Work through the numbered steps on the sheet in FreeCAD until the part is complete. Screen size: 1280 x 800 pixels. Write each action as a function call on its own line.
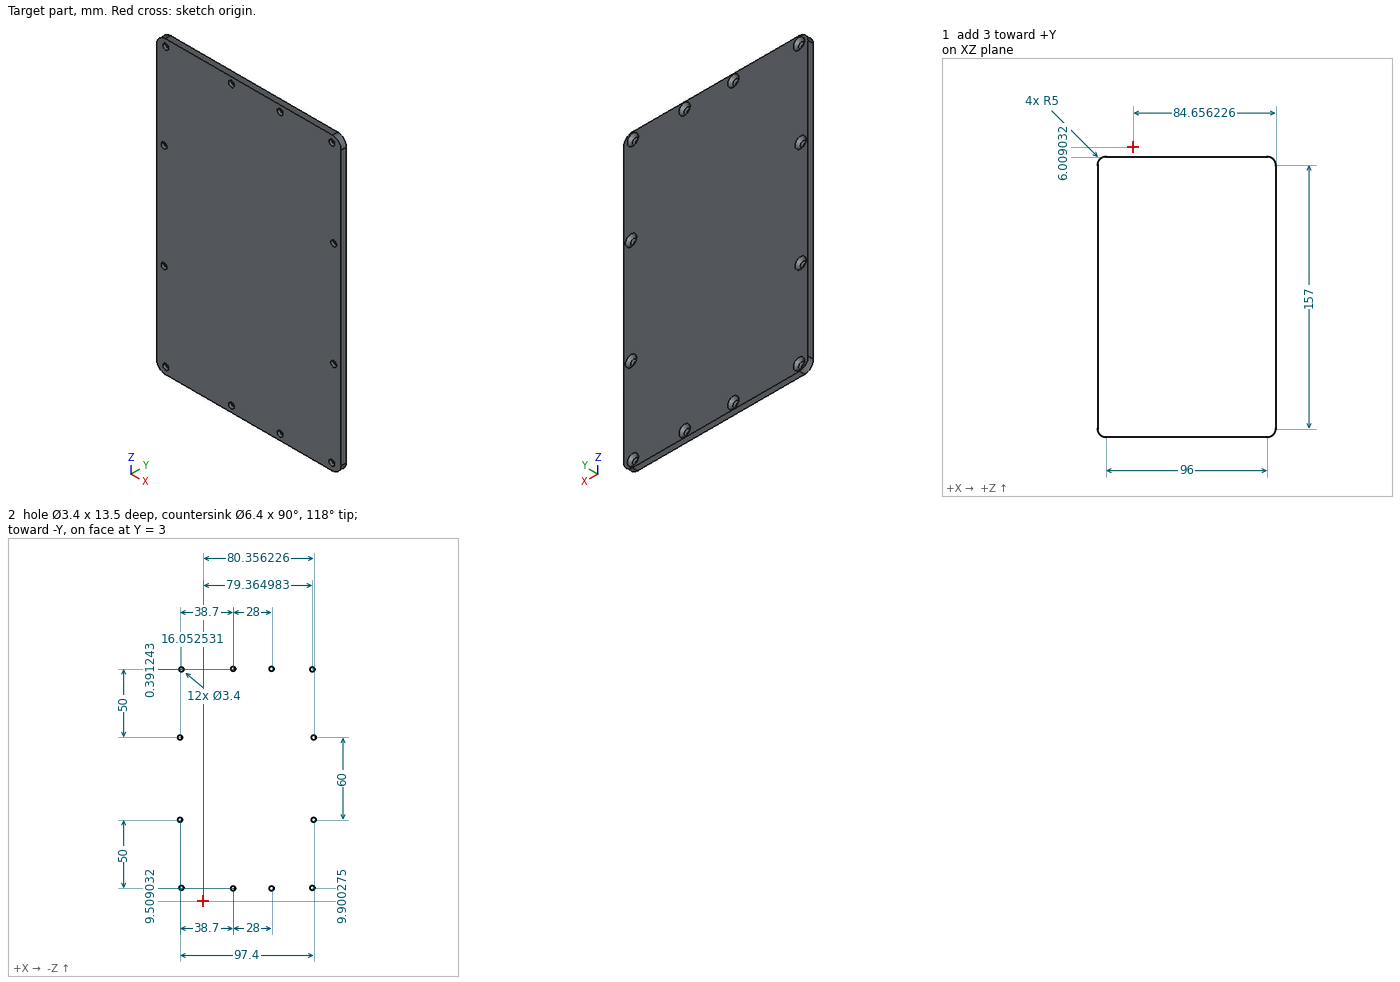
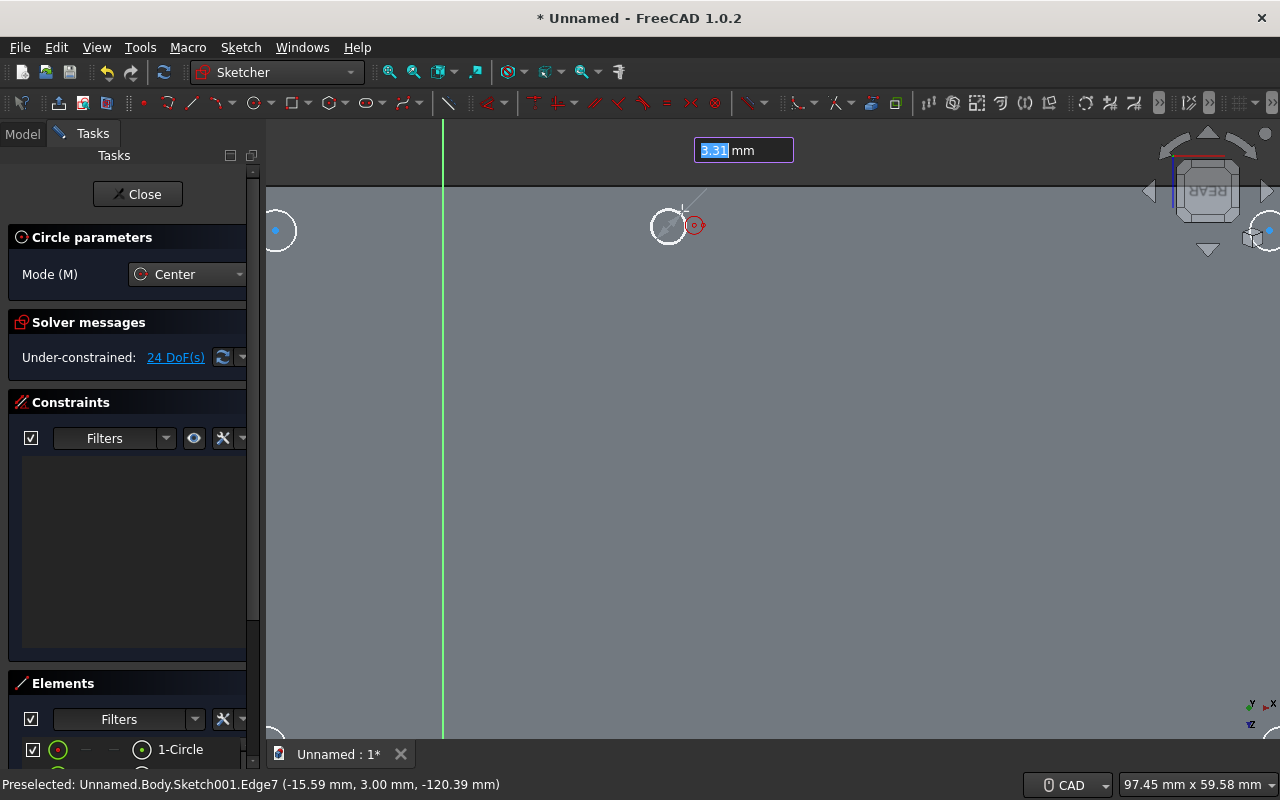
click(681, 209)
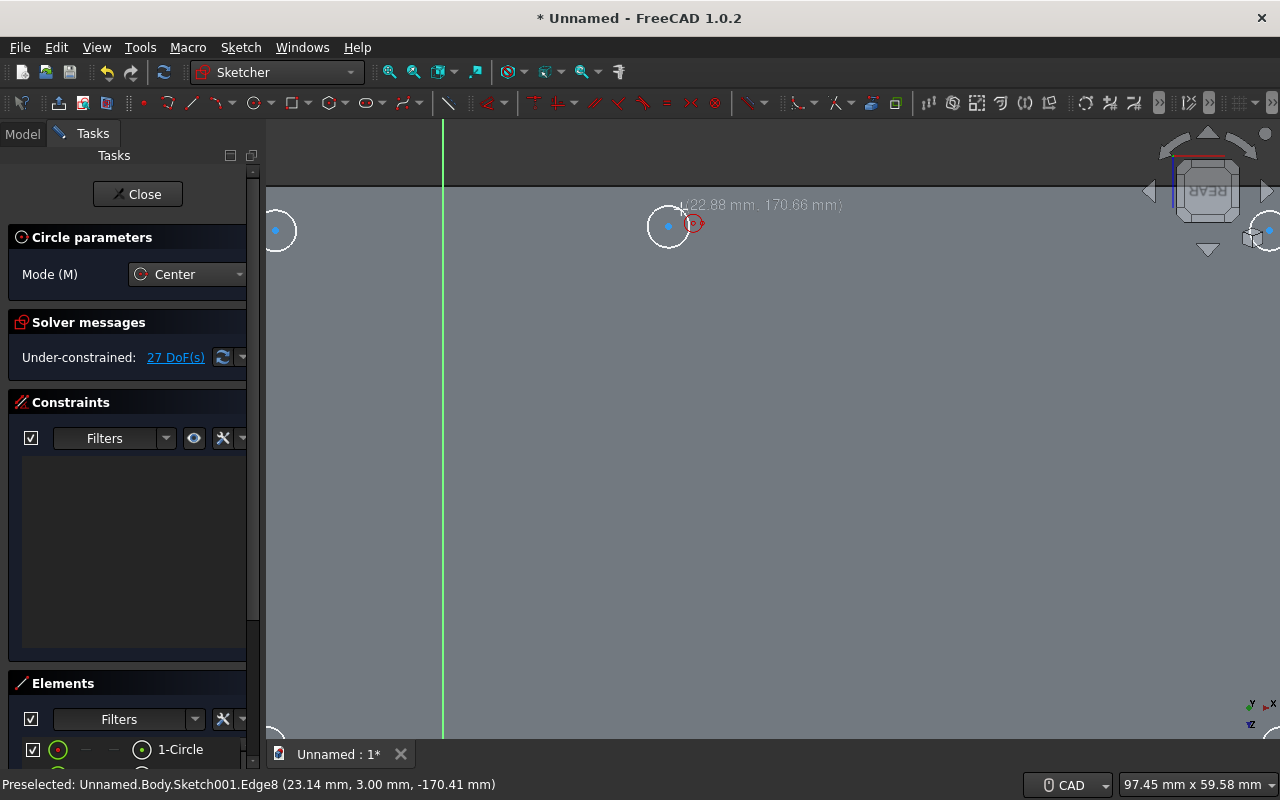
scroll(960, 222, up, 2)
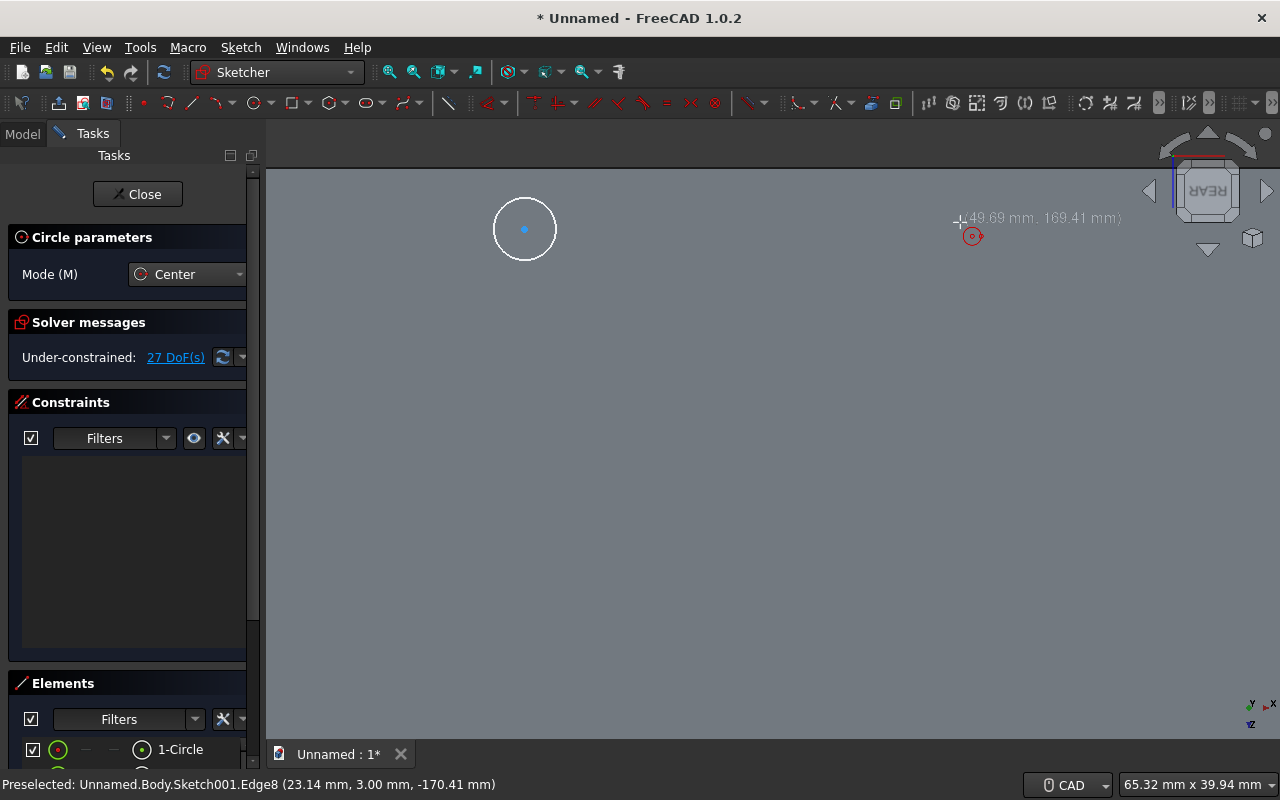
scroll(709, 212, down, 9)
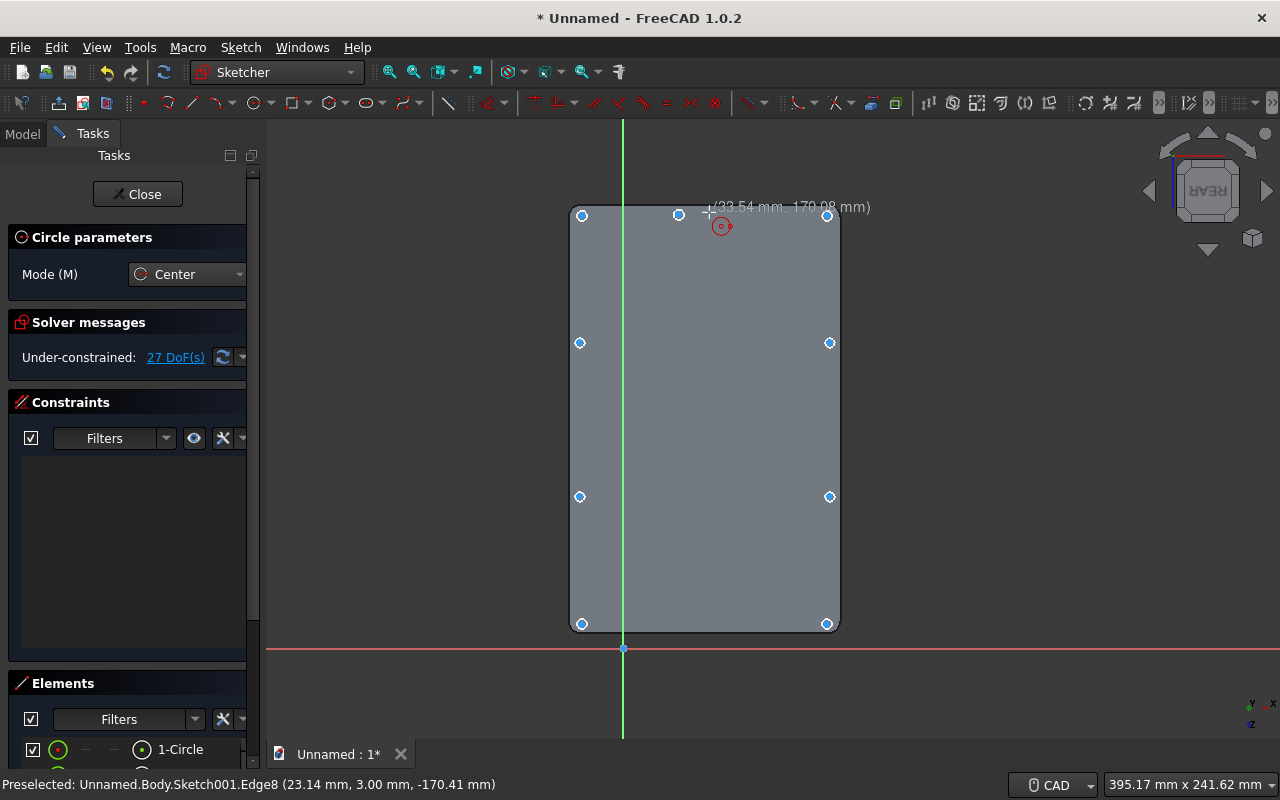
click(751, 214)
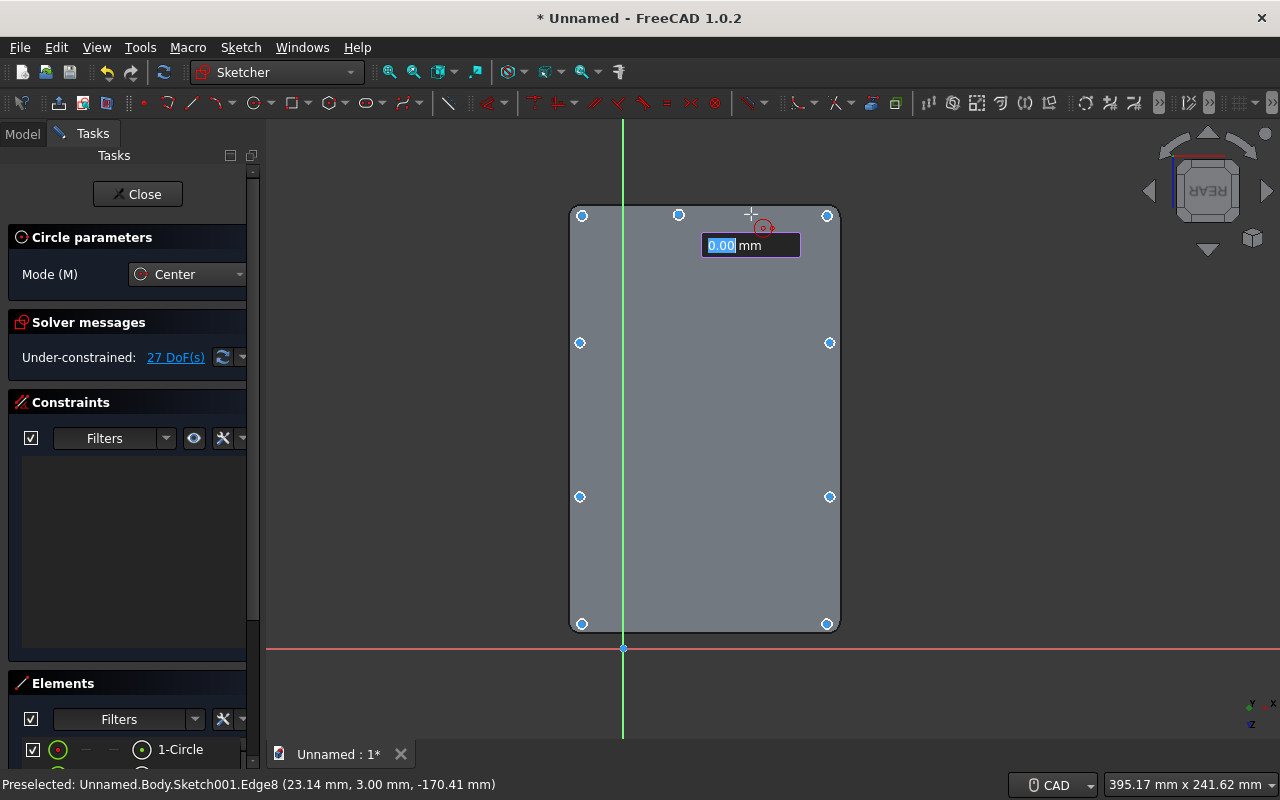
scroll(754, 211, up, 7)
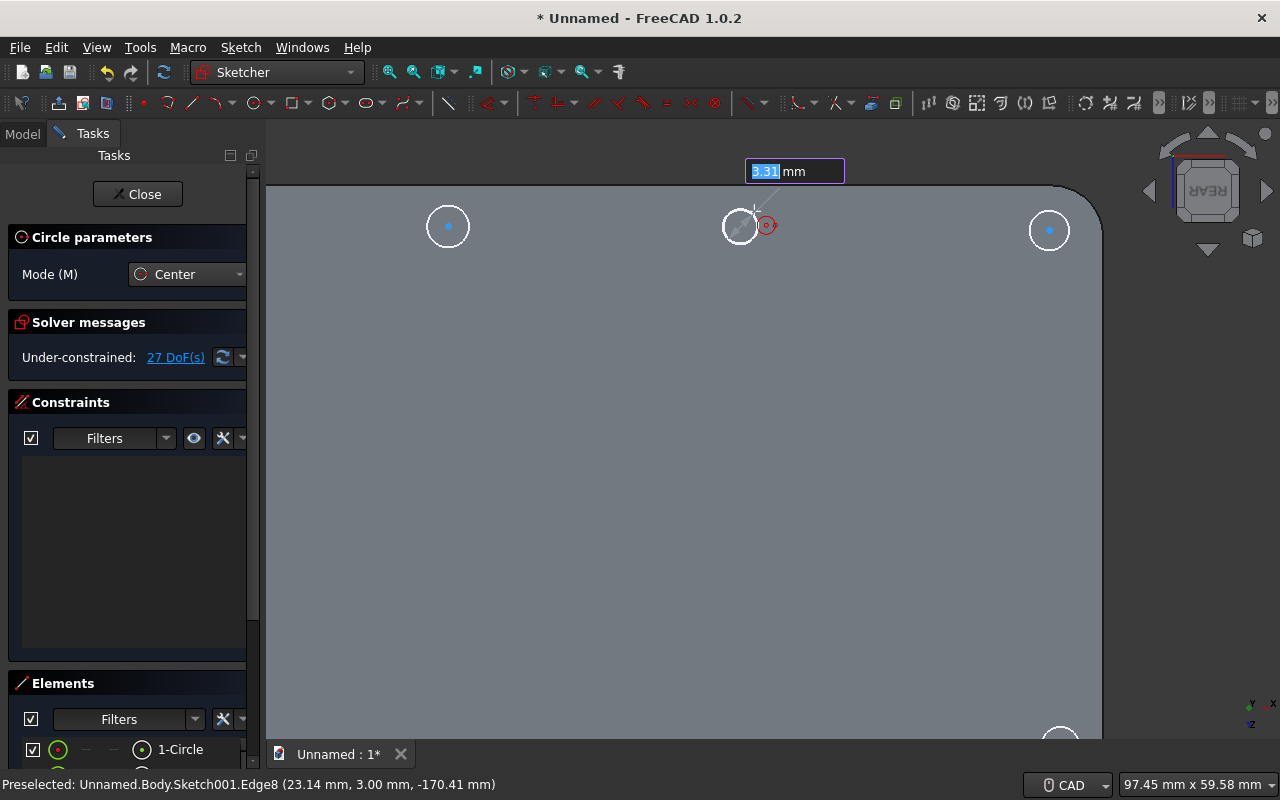
click(752, 209)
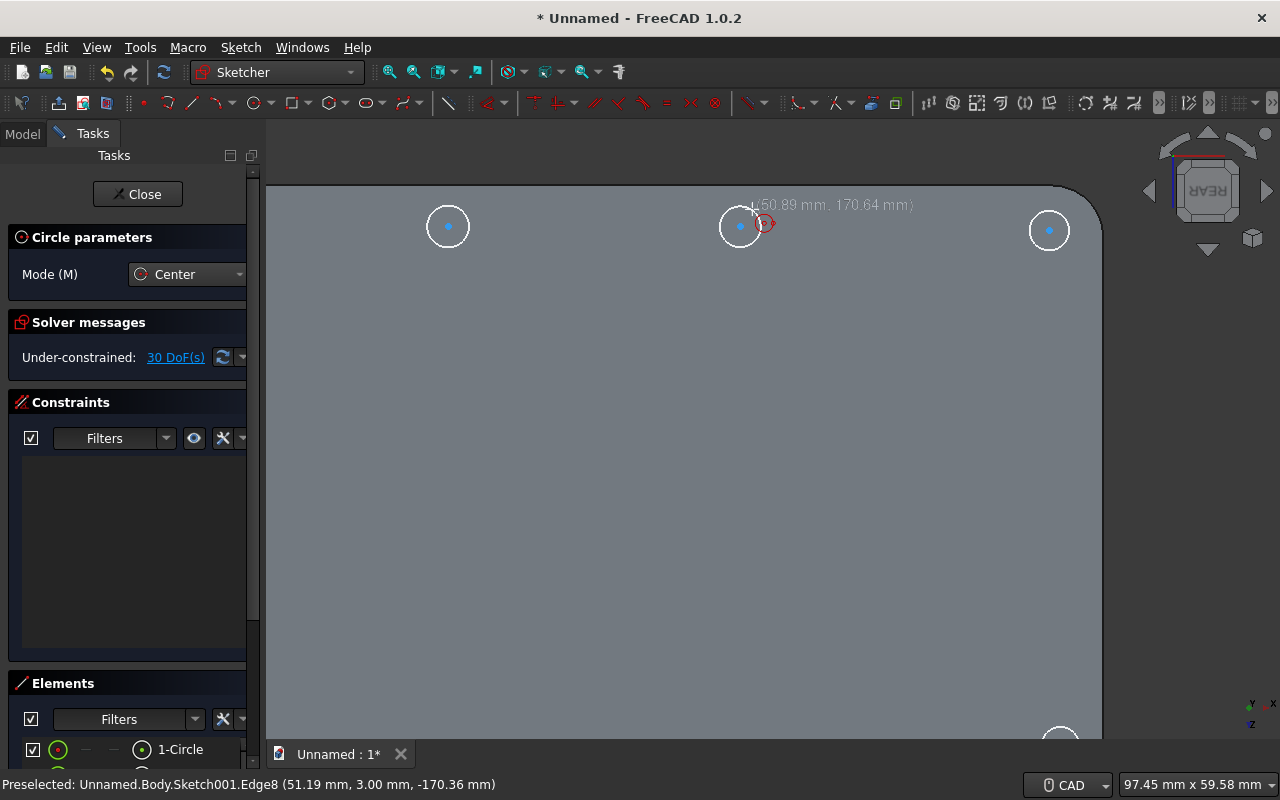
scroll(754, 211, down, 7)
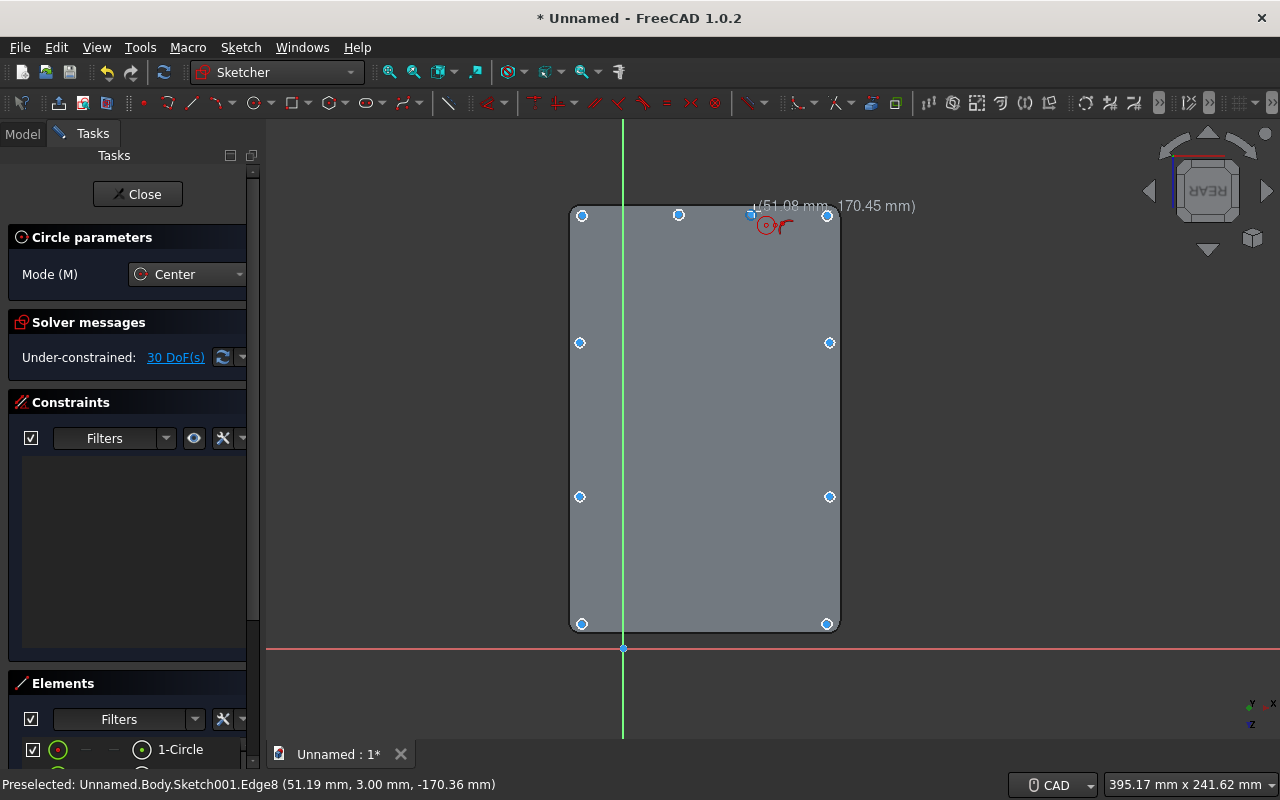
scroll(679, 624, up, 9)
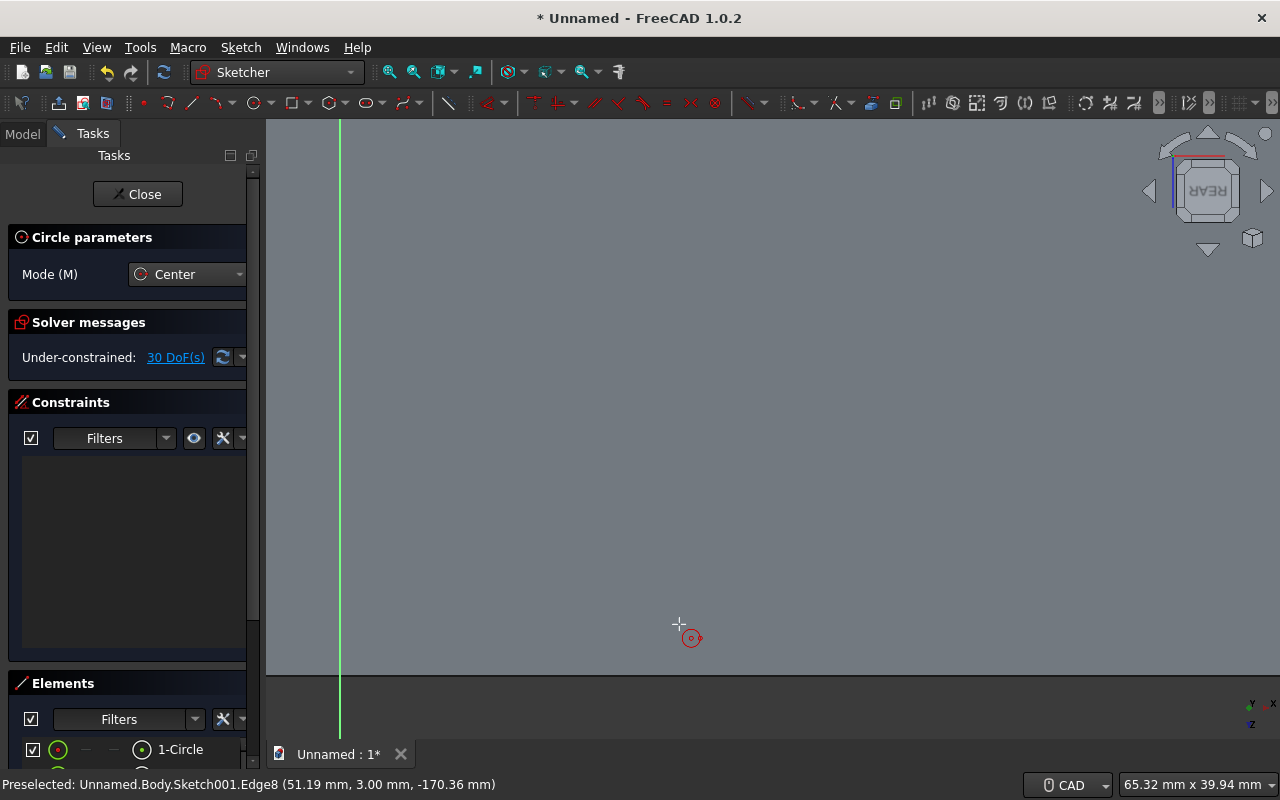
scroll(679, 625, down, 9)